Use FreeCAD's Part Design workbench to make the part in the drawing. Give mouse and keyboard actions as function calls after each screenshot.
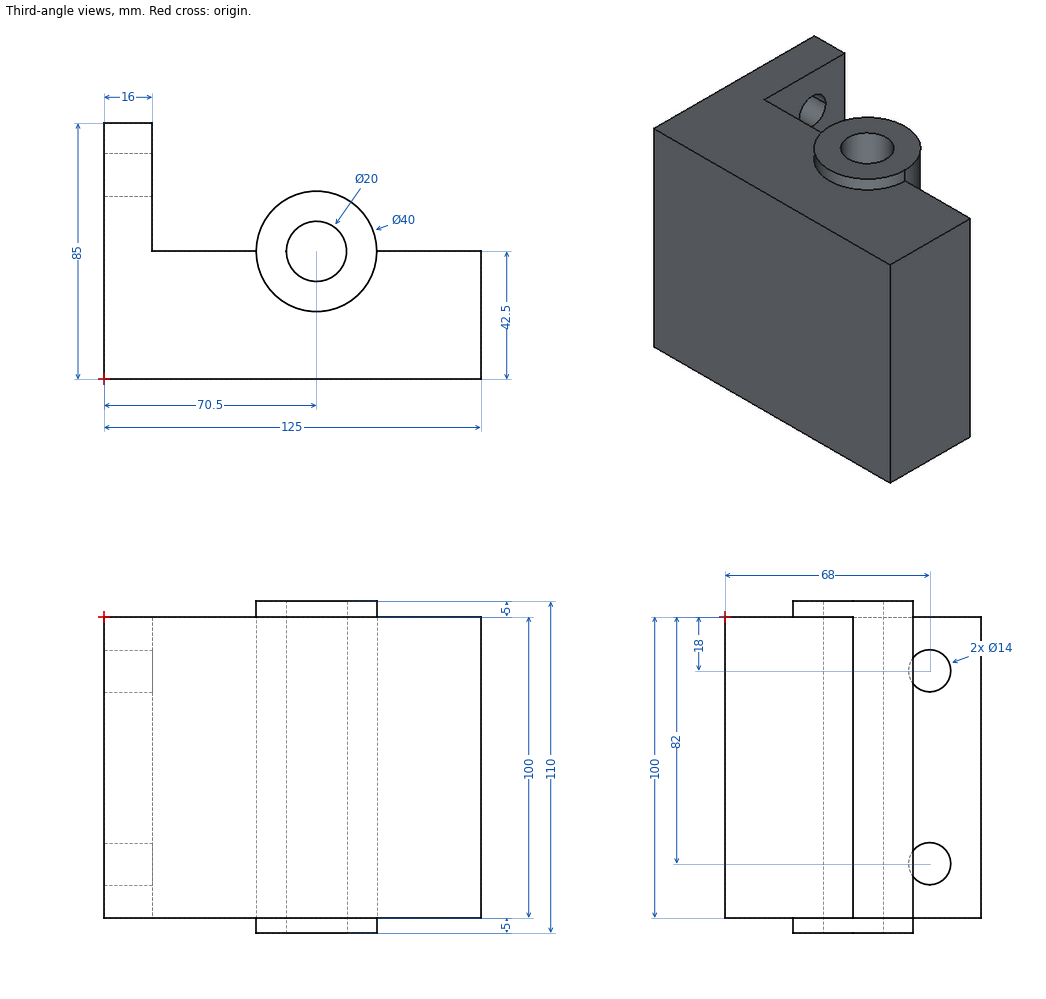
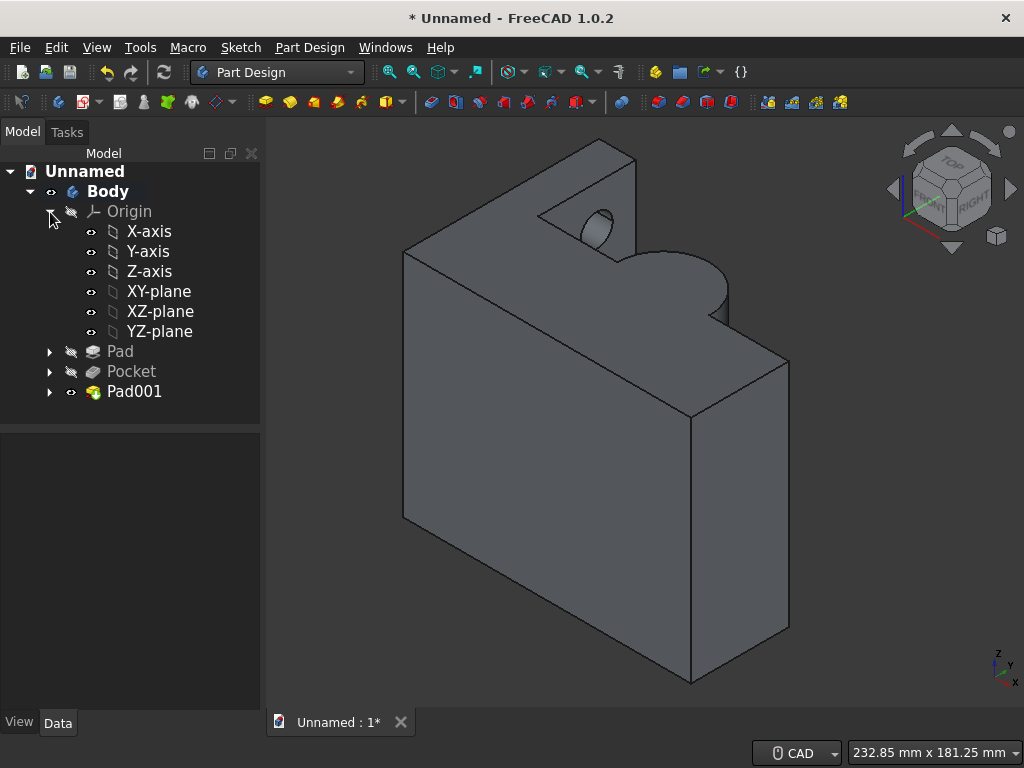
click(136, 292)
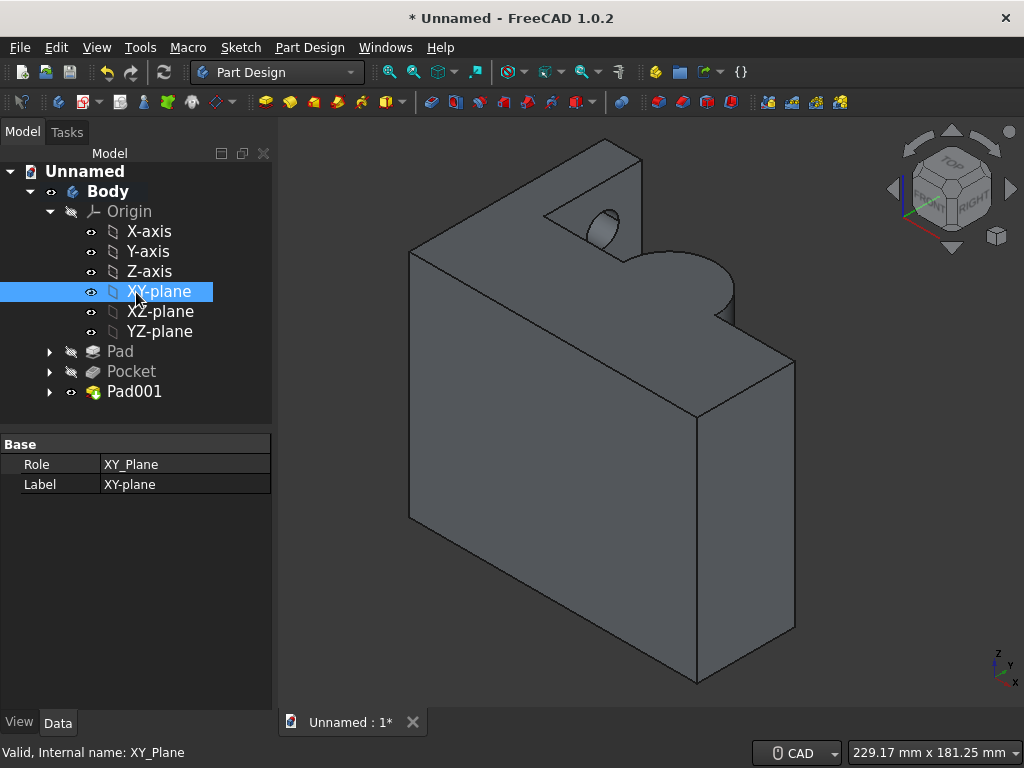
click(216, 102)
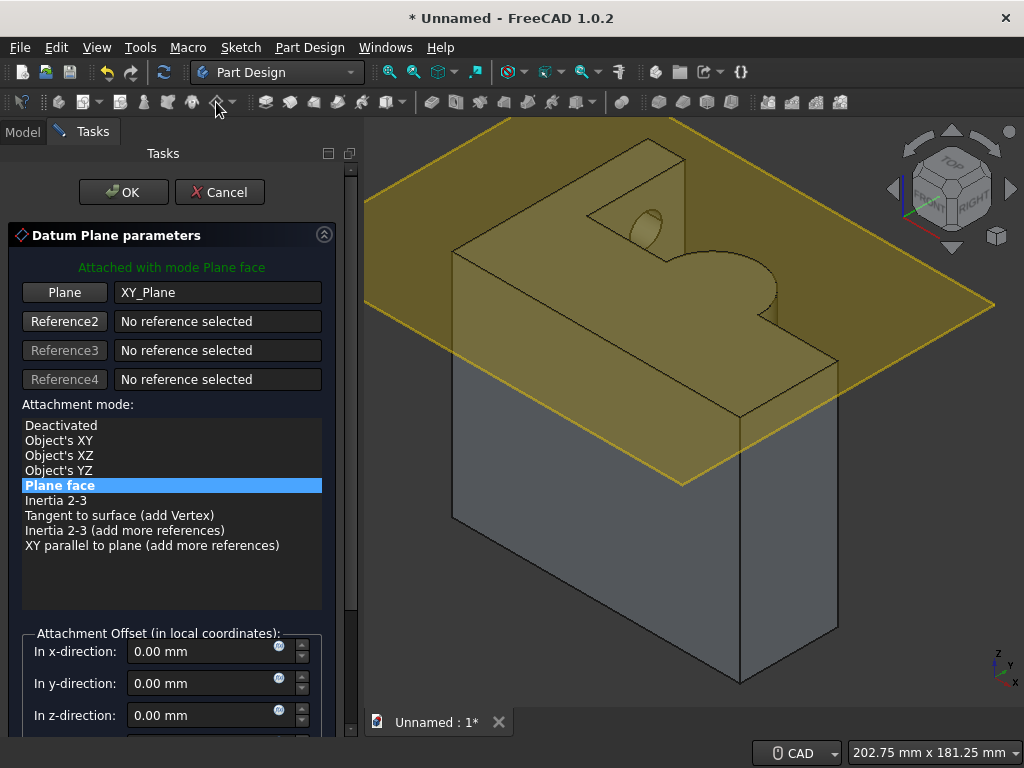
triple_click(210, 715)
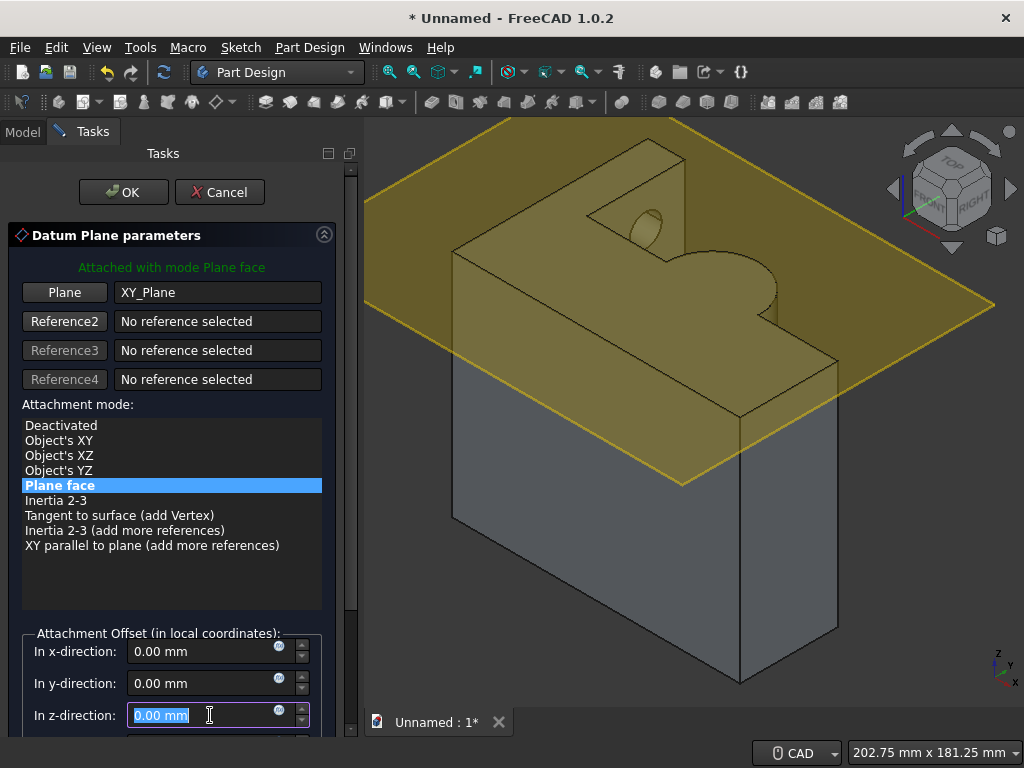
text(5)
key(Tab)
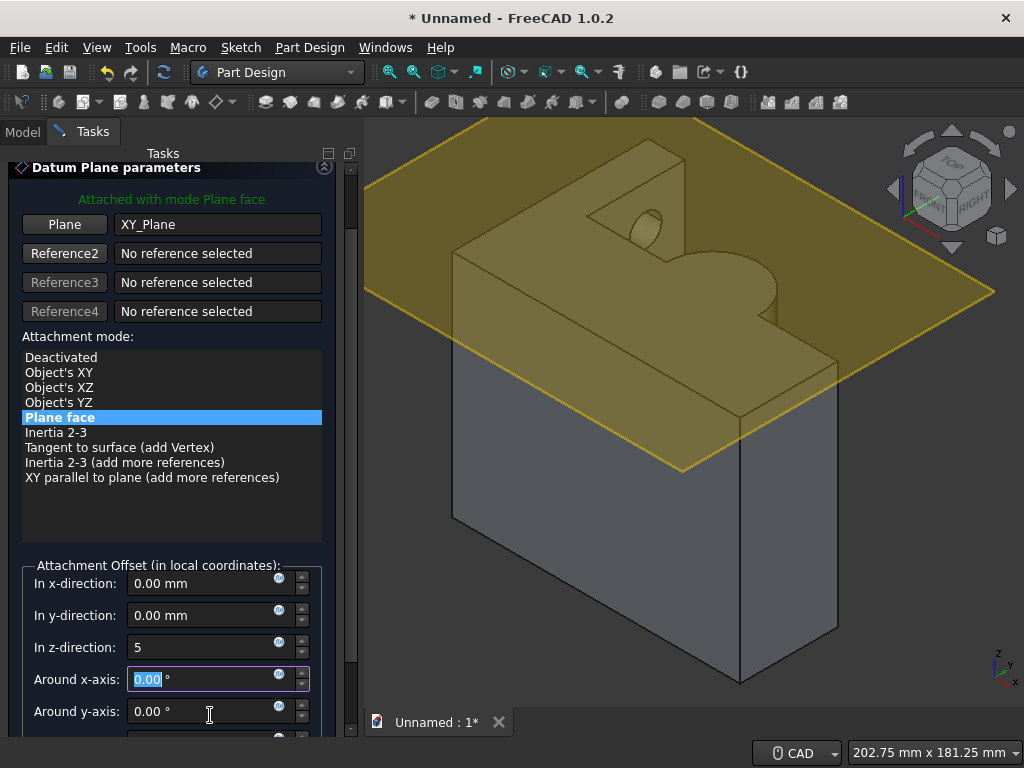
scroll(351, 450, up, 2)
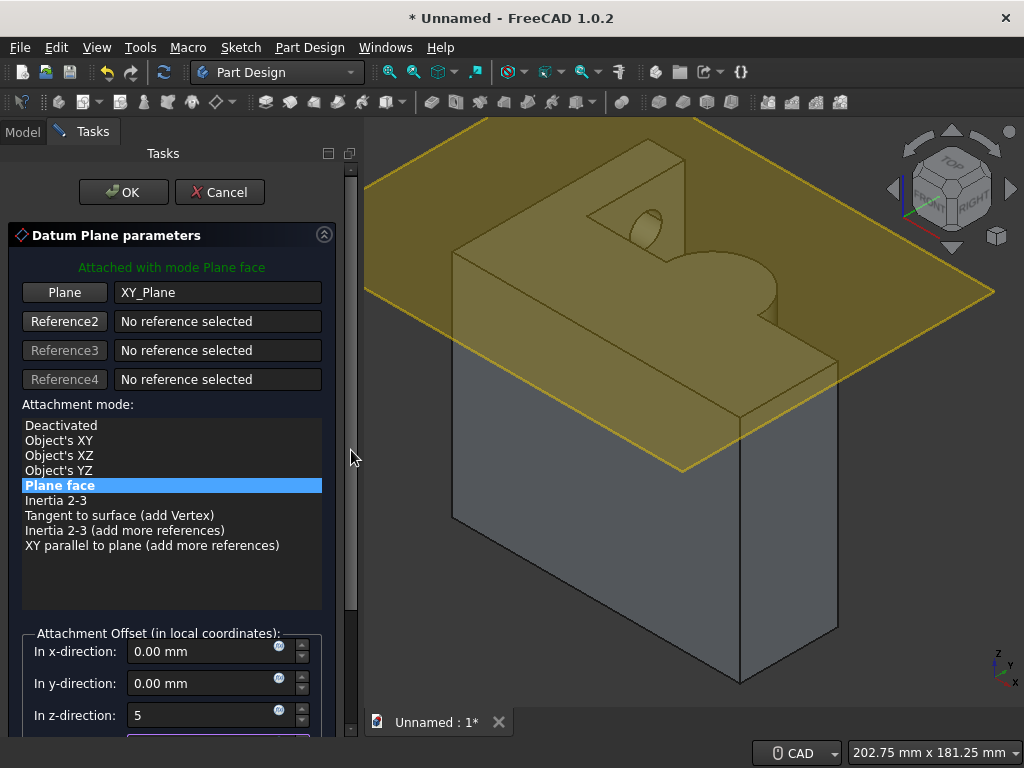
click(124, 192)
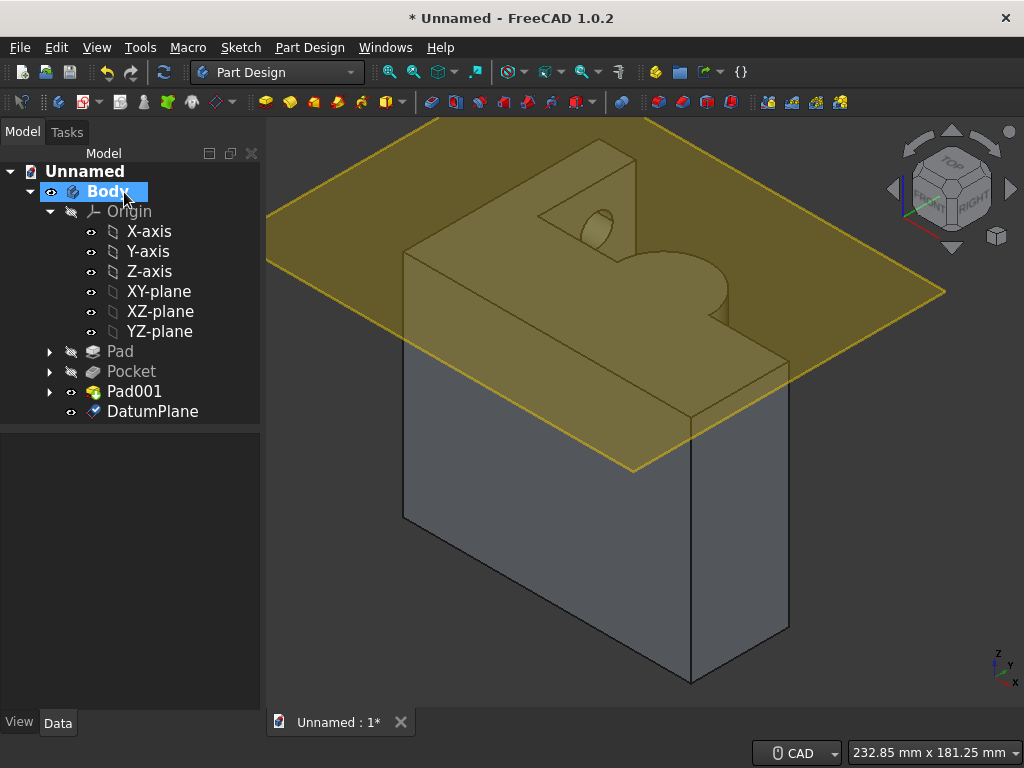
click(116, 412)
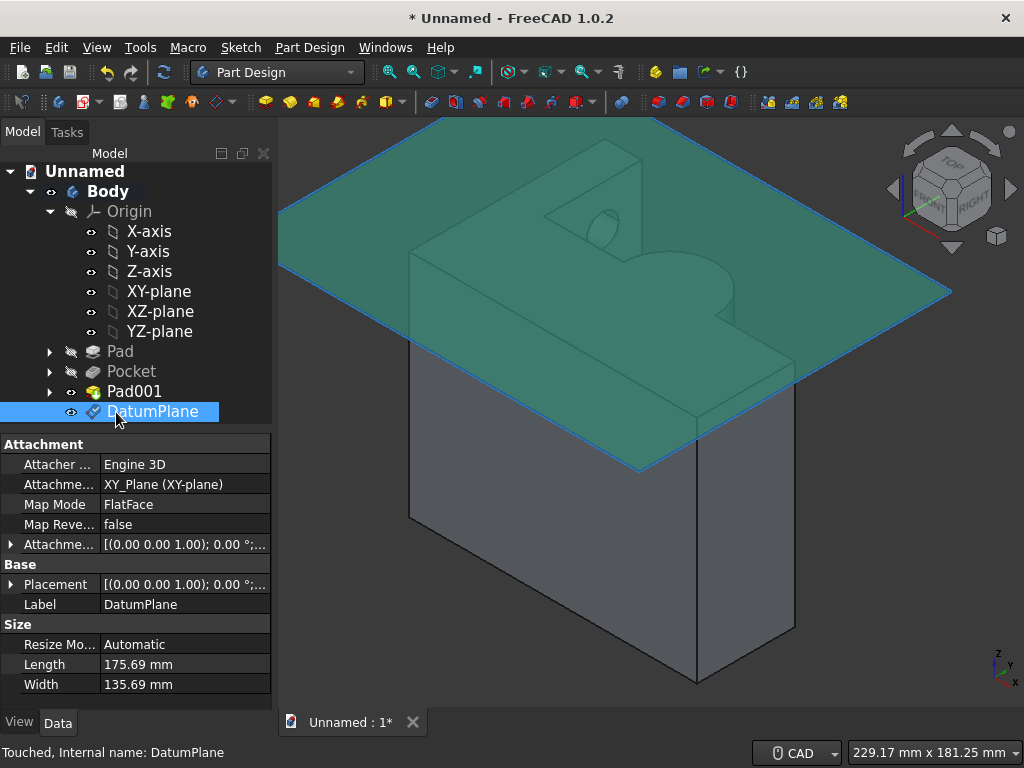
click(84, 102)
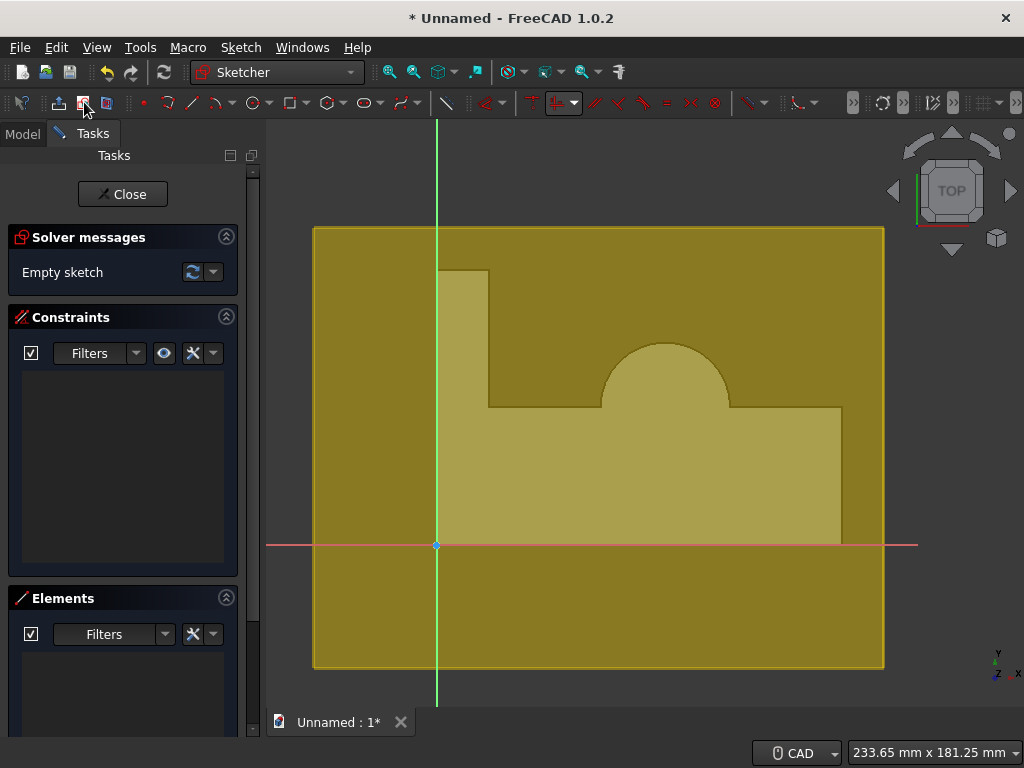
scroll(598, 507, up, 2)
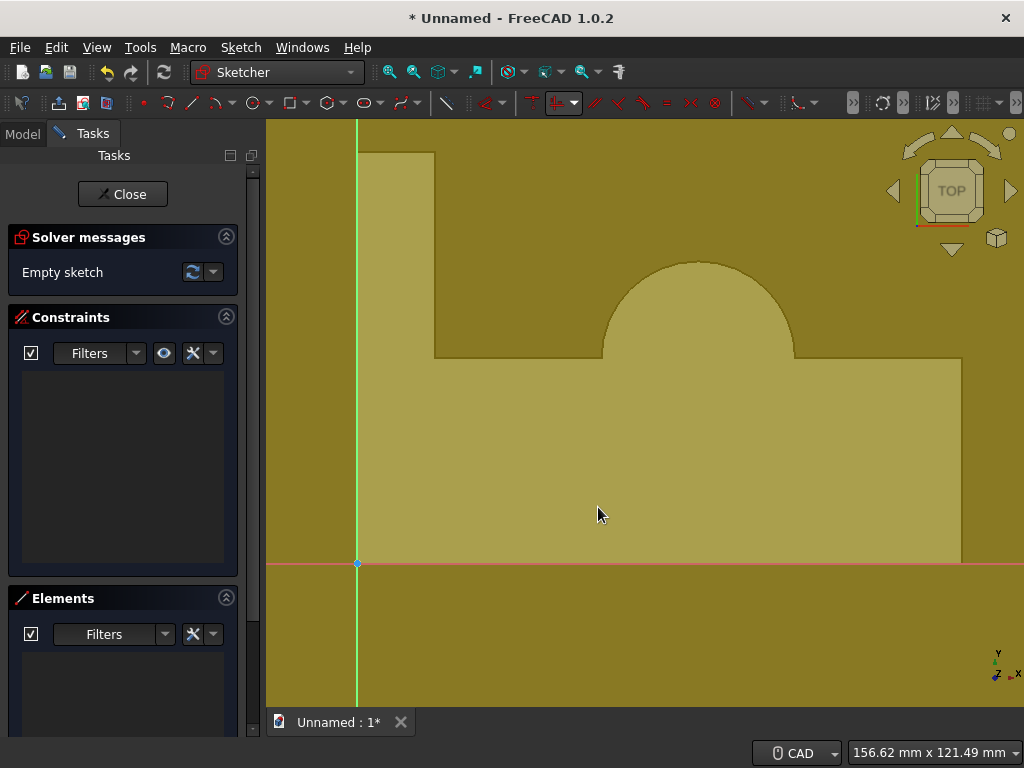
click(254, 104)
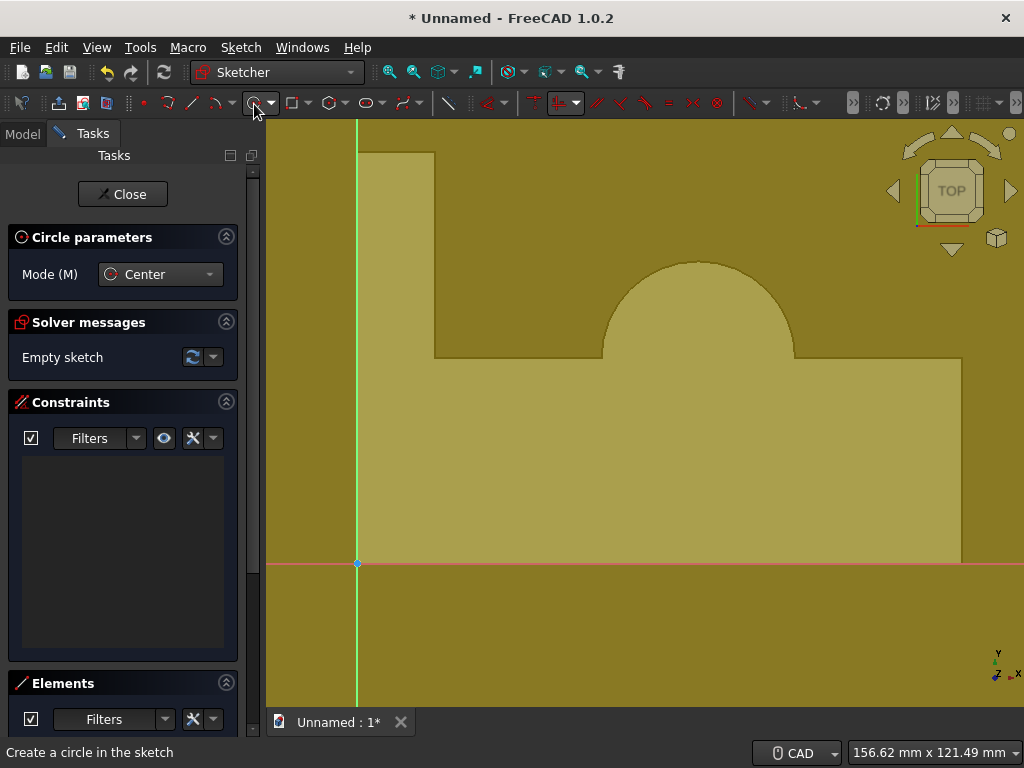
click(698, 358)
move(767, 290)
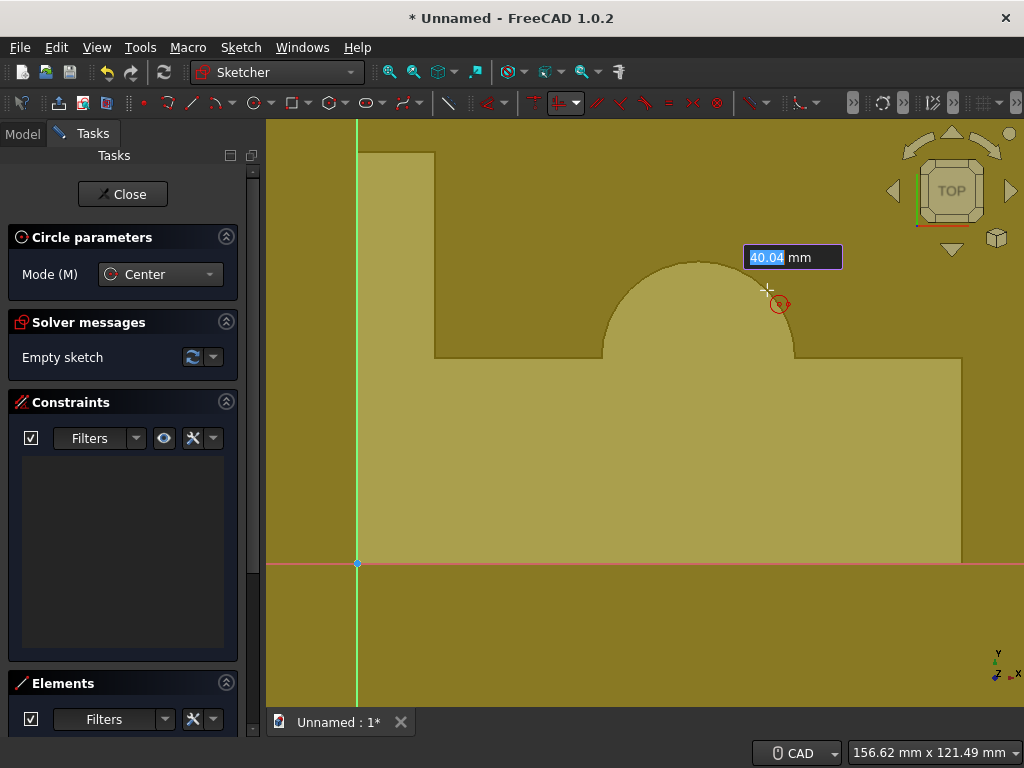
text(40)
key(Return)
key(Escape)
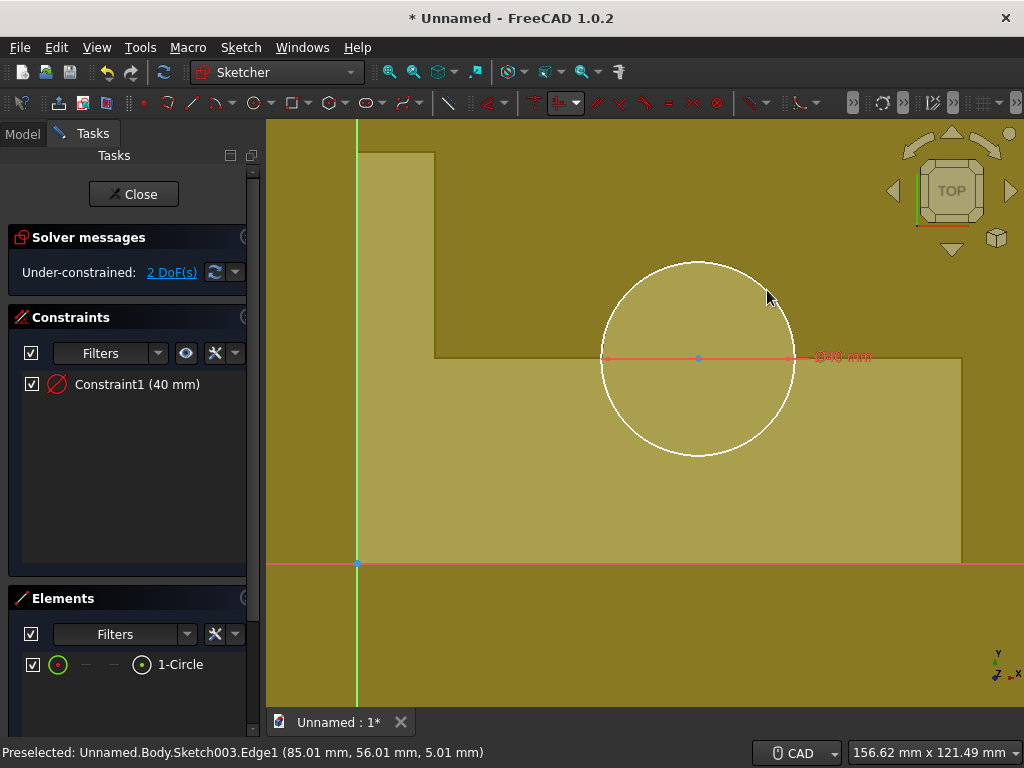
click(488, 104)